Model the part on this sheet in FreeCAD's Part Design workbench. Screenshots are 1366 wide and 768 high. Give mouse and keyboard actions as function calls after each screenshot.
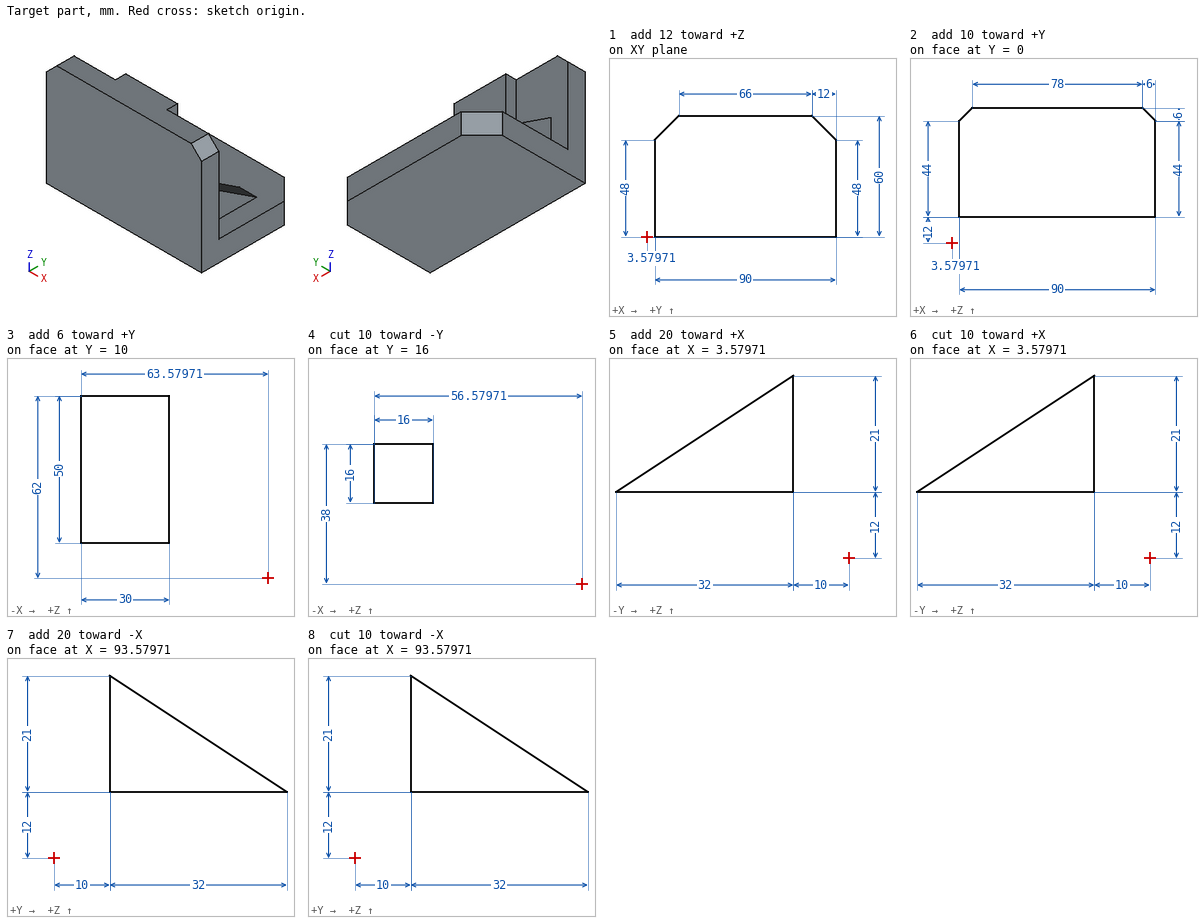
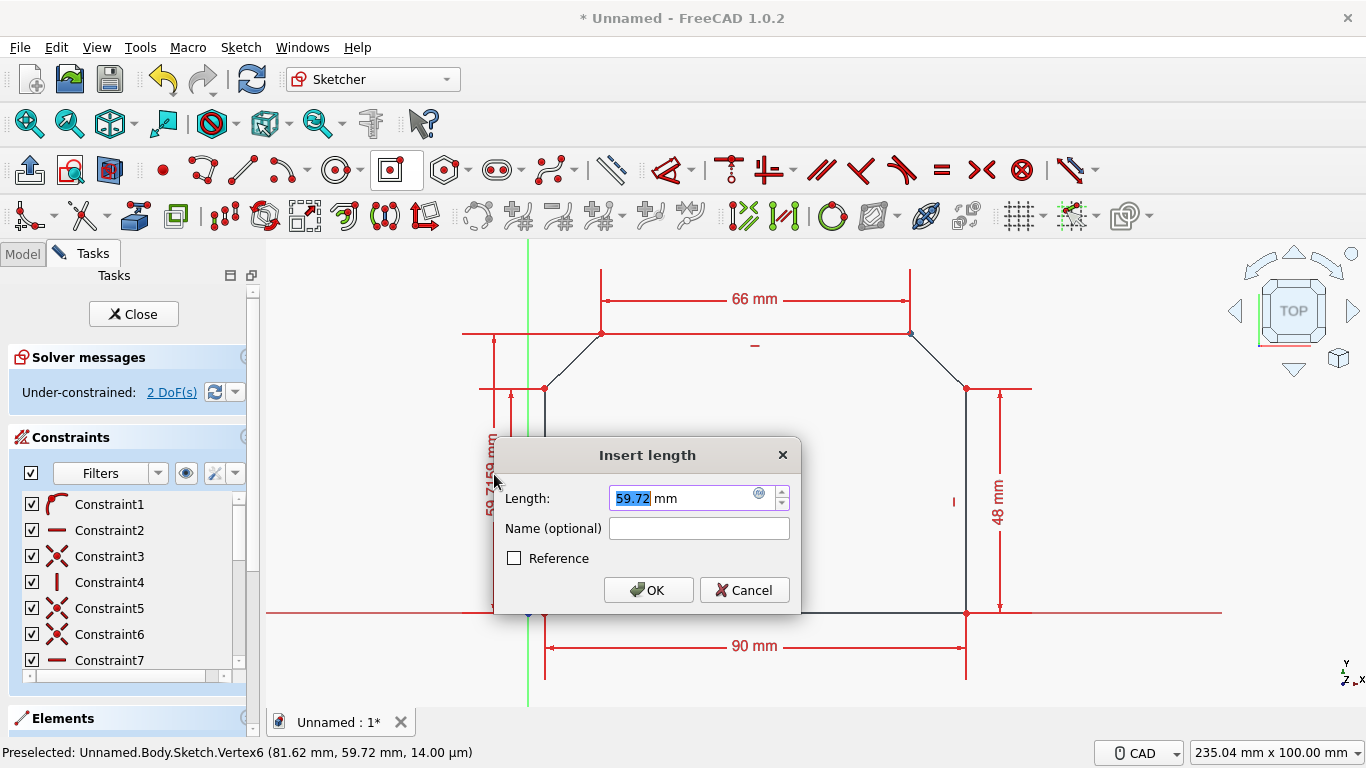
text(60)
key(Return)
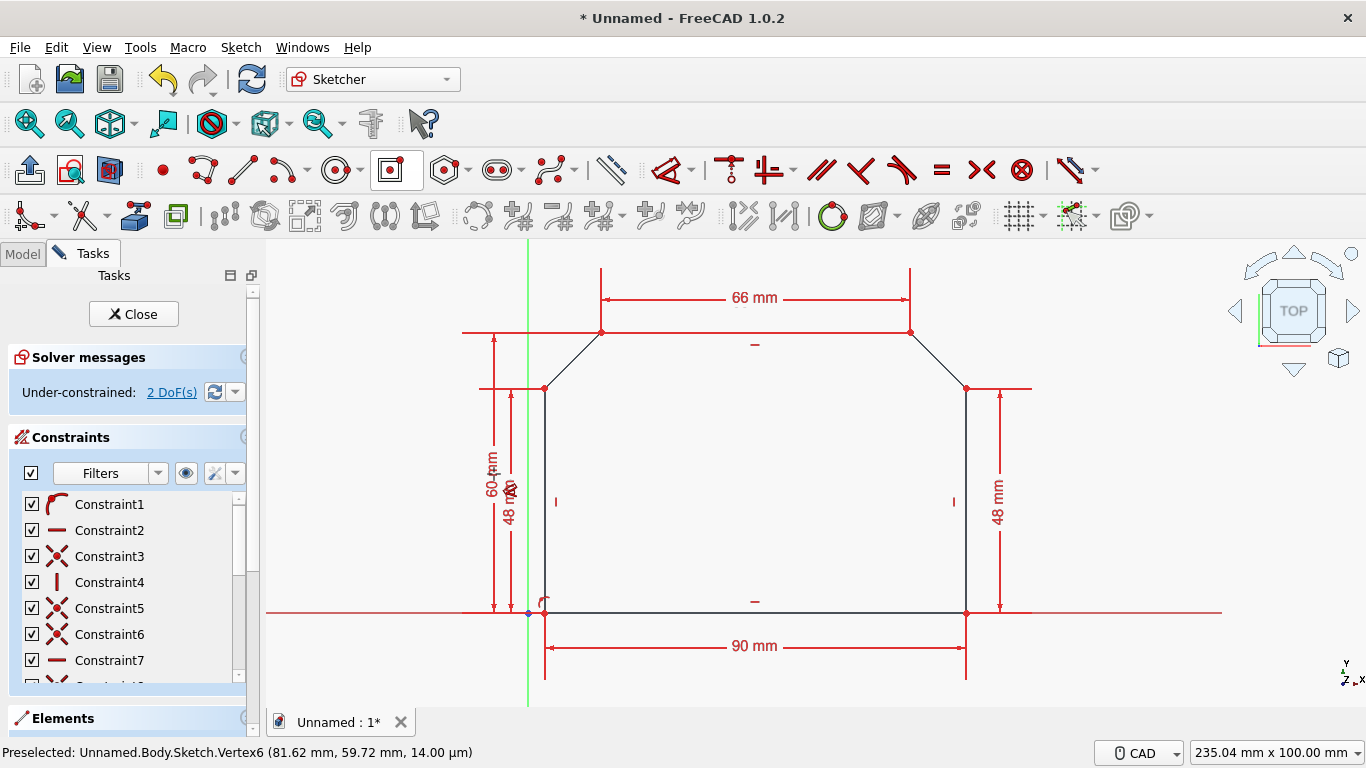
click(949, 372)
click(938, 299)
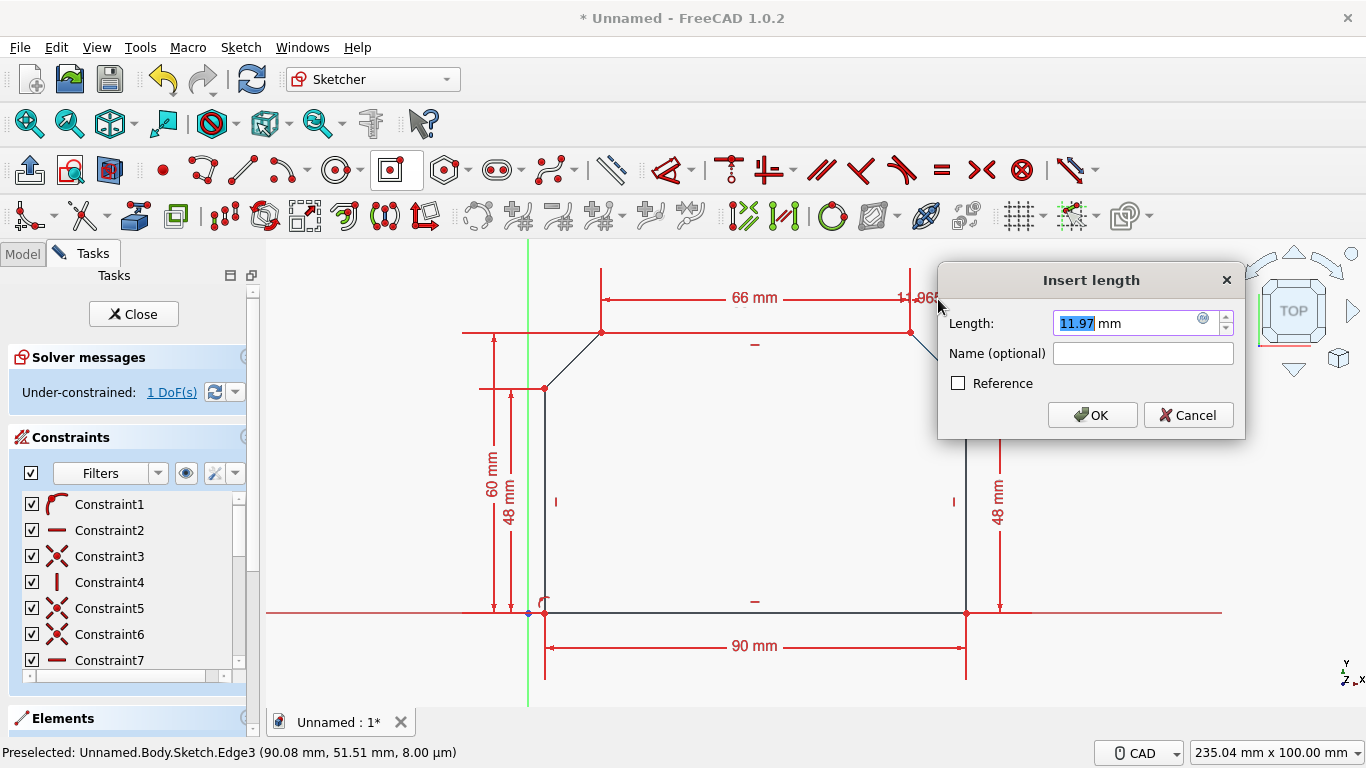
text(12)
key(Return)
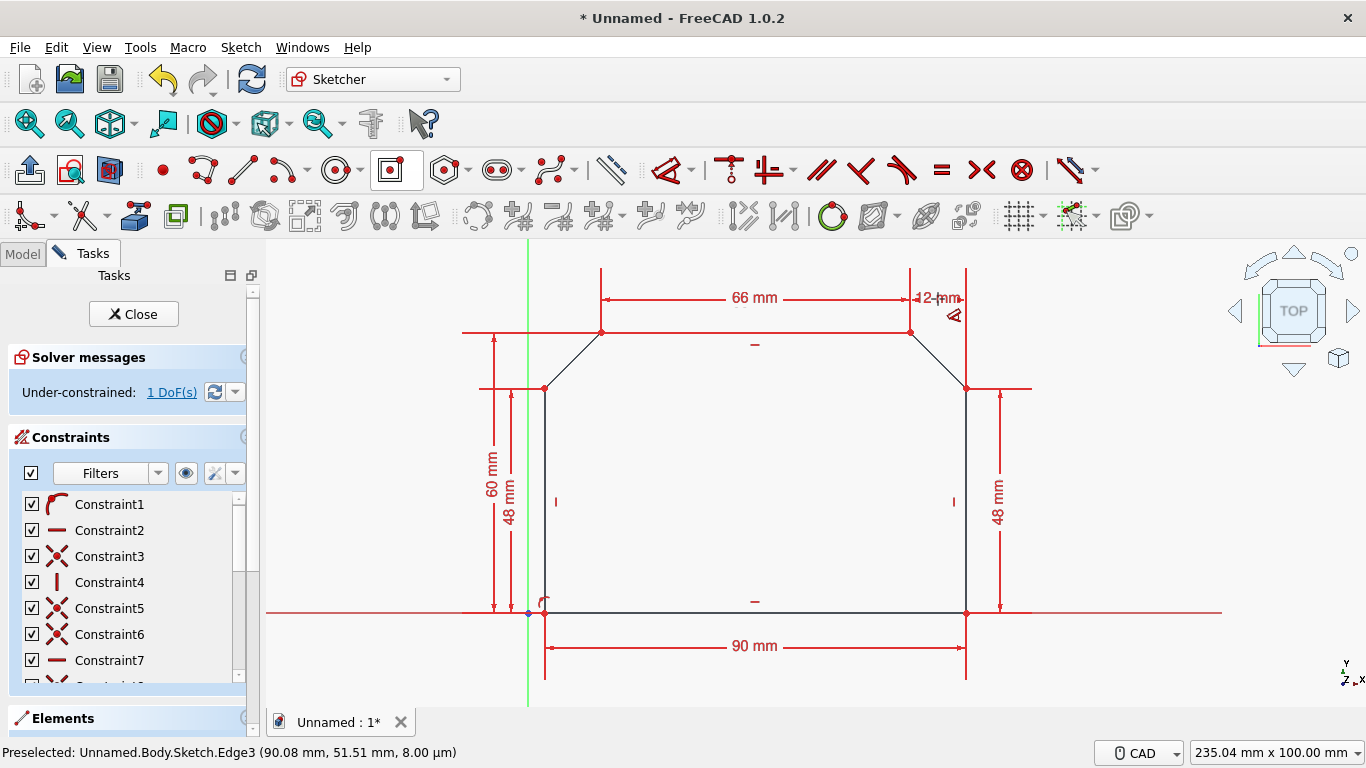
scroll(545, 613, up, 5)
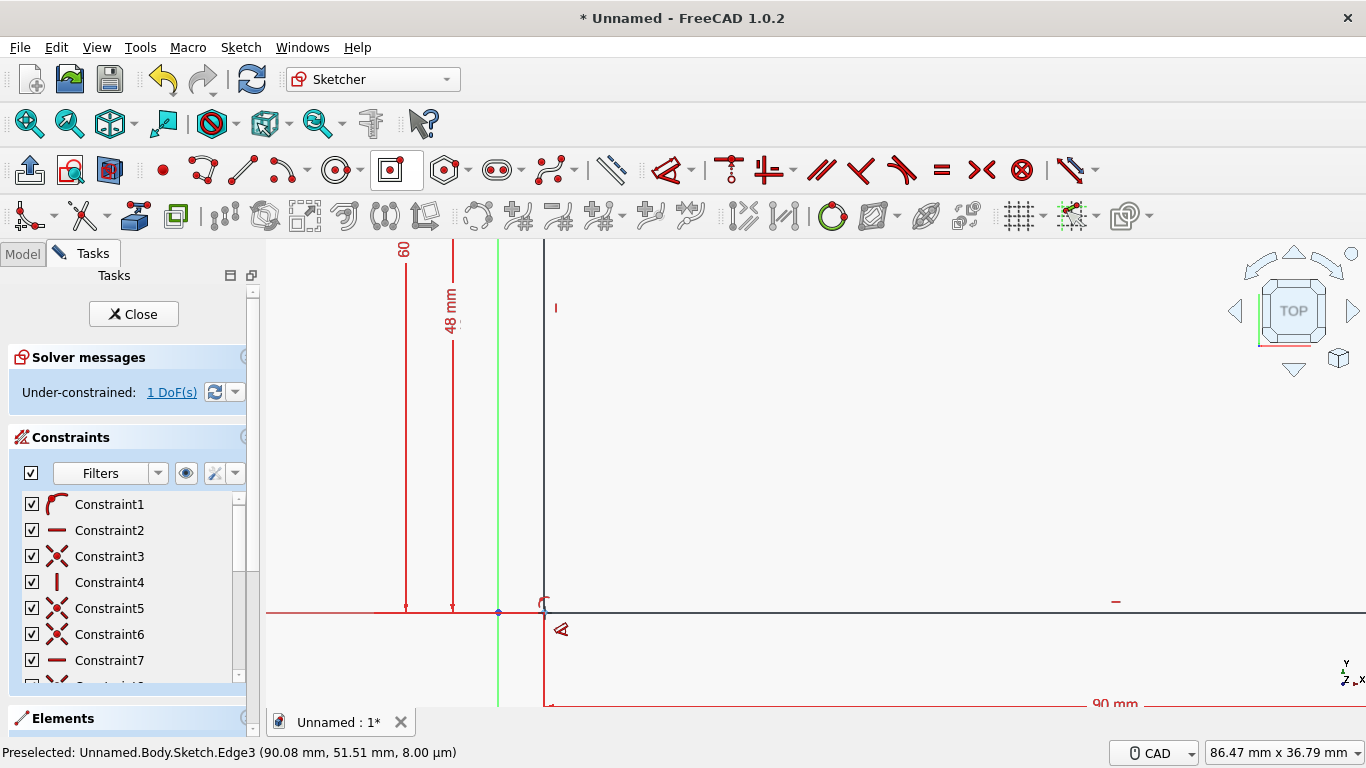
click(544, 613)
click(521, 647)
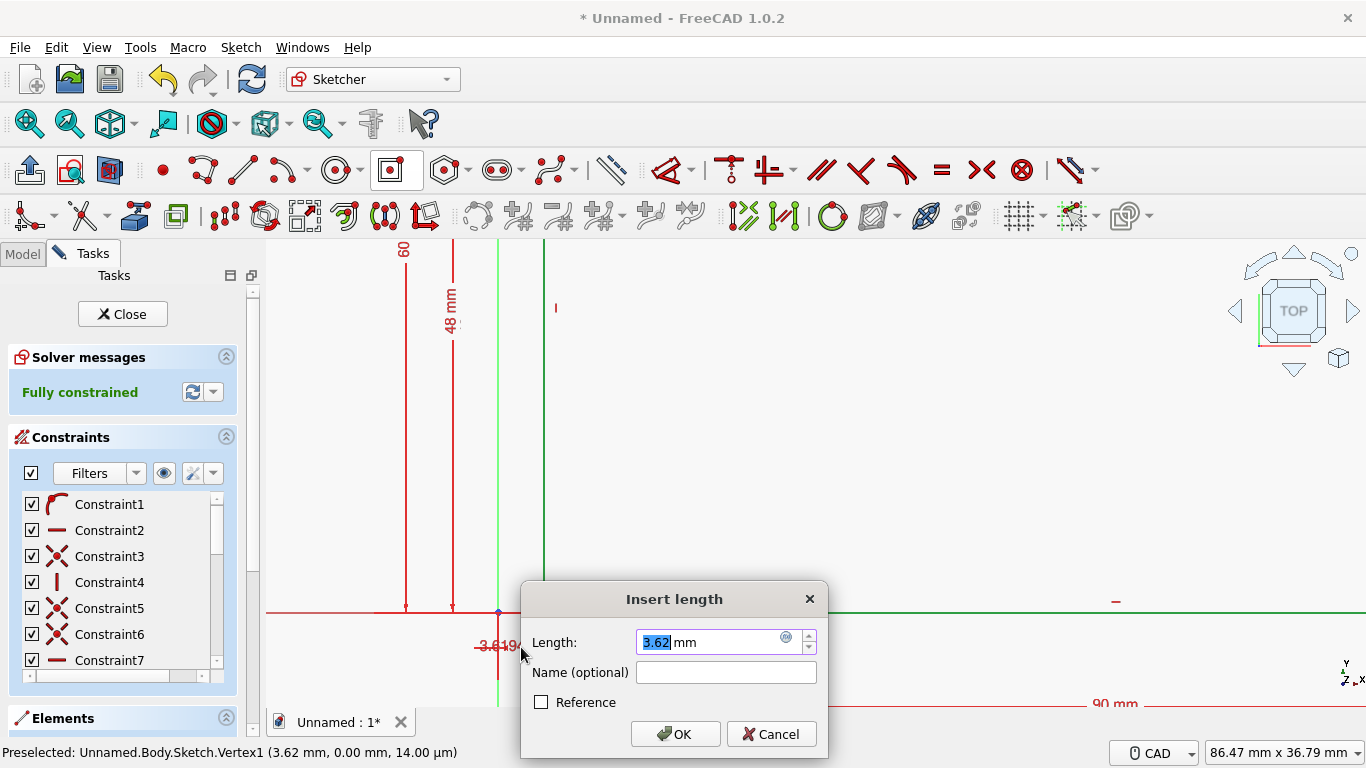
text(3.57971)
key(Return)
key(Escape)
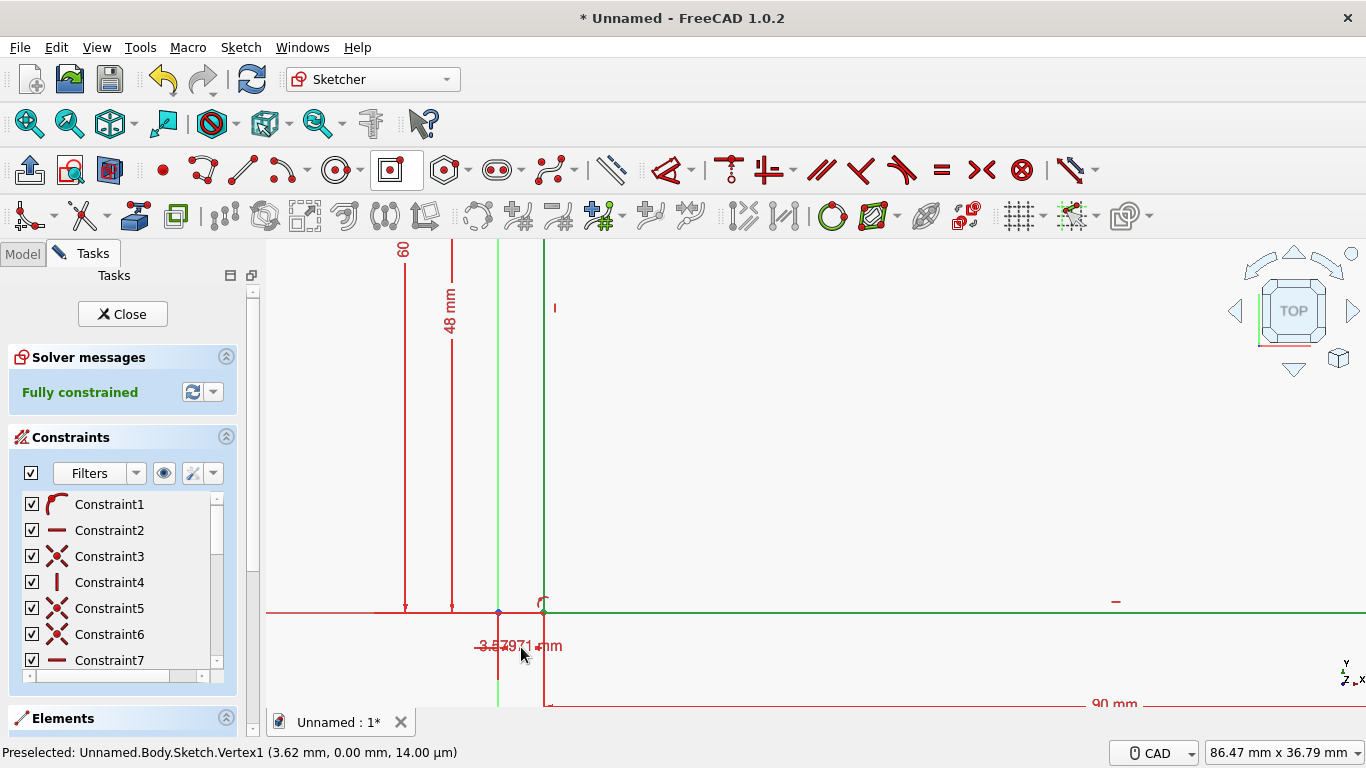
click(123, 314)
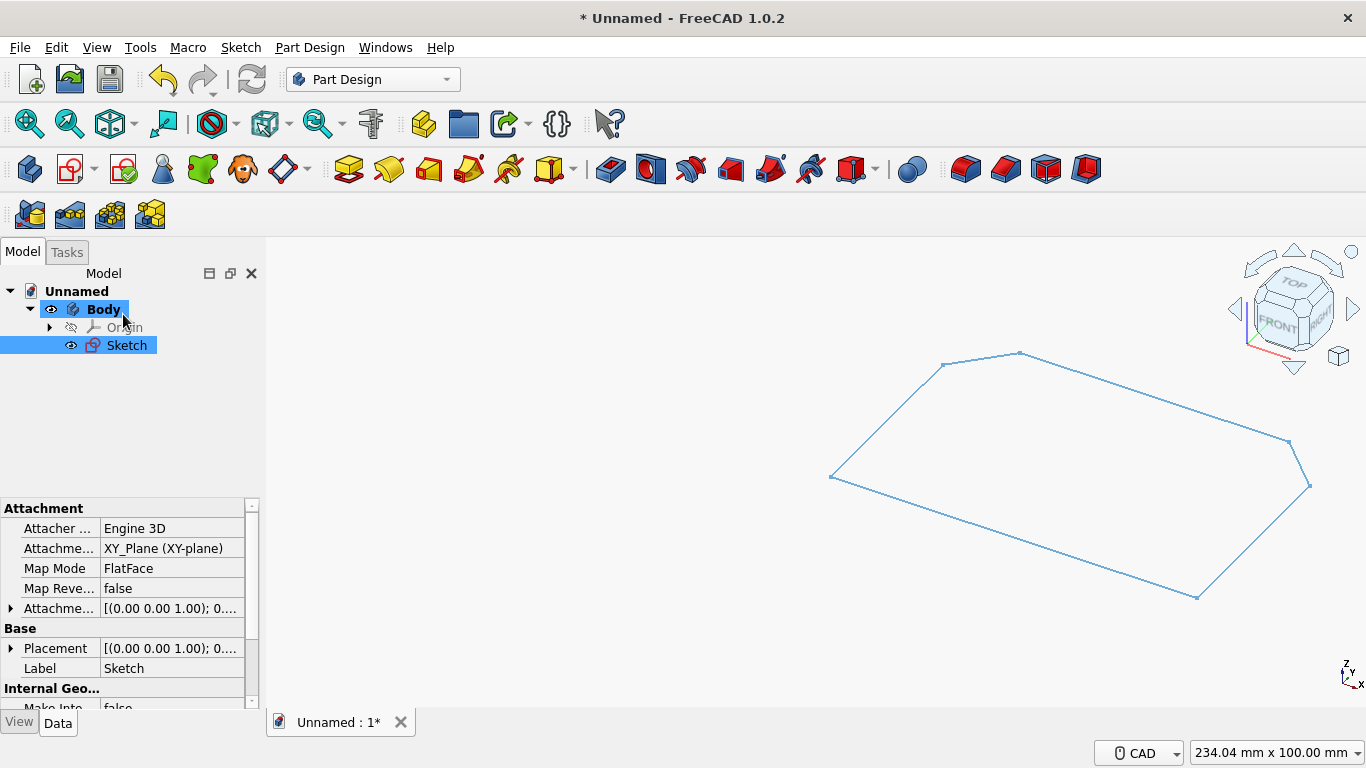
click(350, 170)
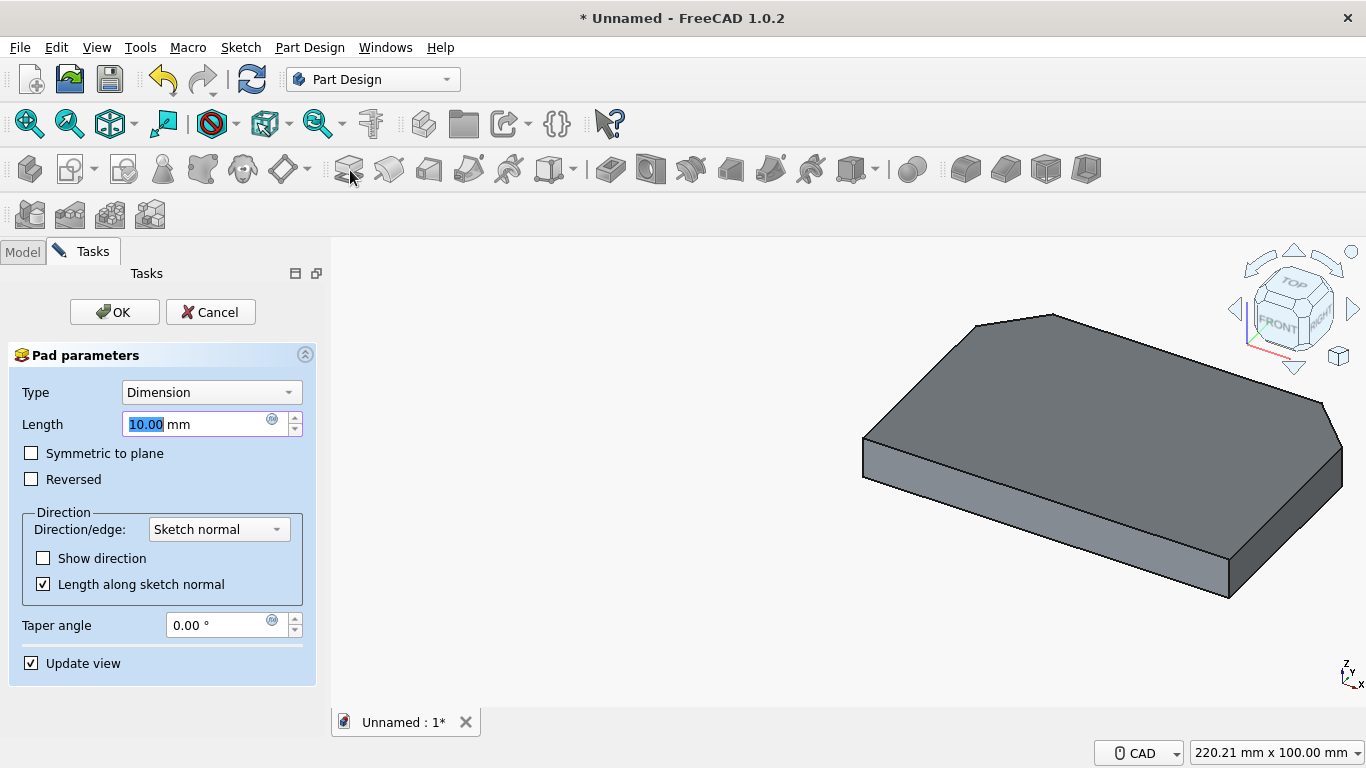
text(12)
key(Tab)